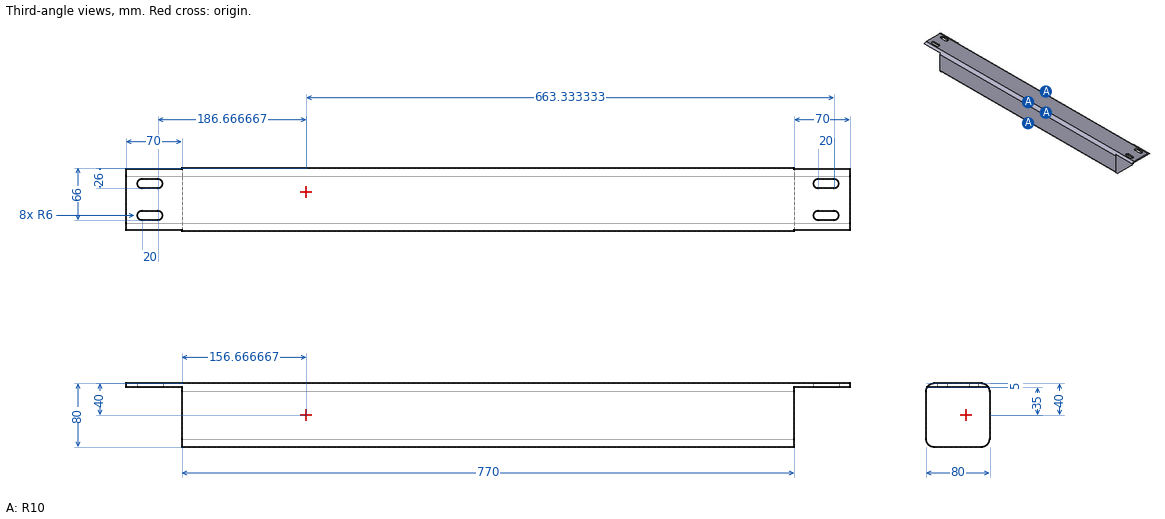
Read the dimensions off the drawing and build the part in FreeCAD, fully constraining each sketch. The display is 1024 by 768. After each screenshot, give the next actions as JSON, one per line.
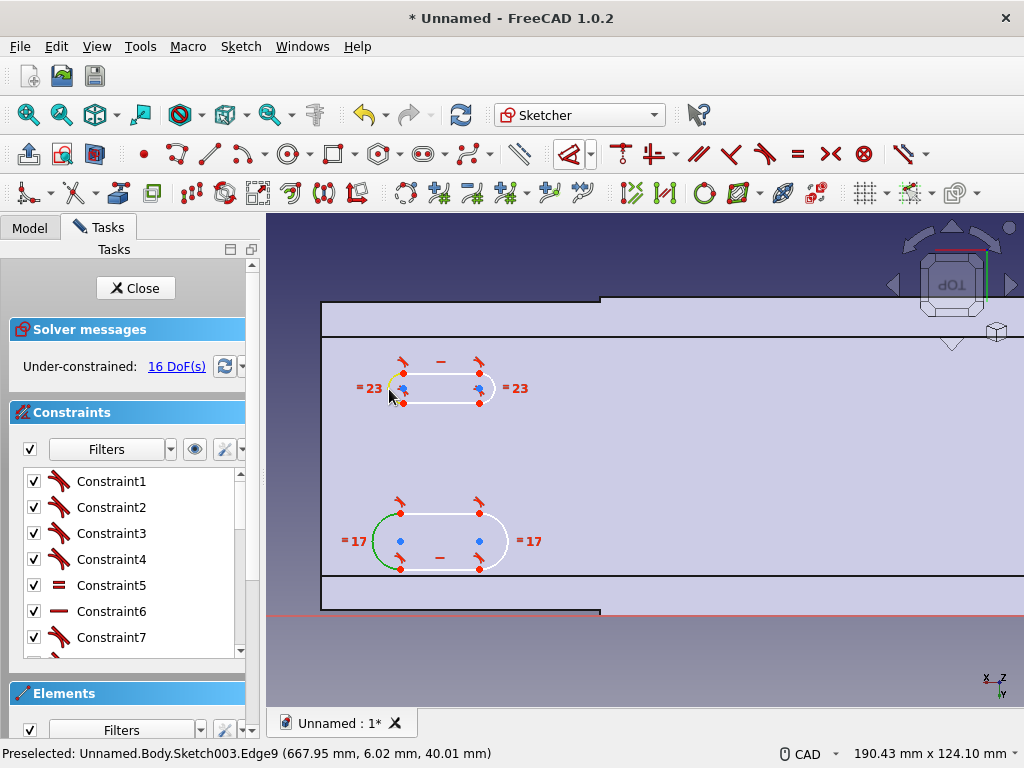
{"action": "left_click", "coordinate": [388, 388]}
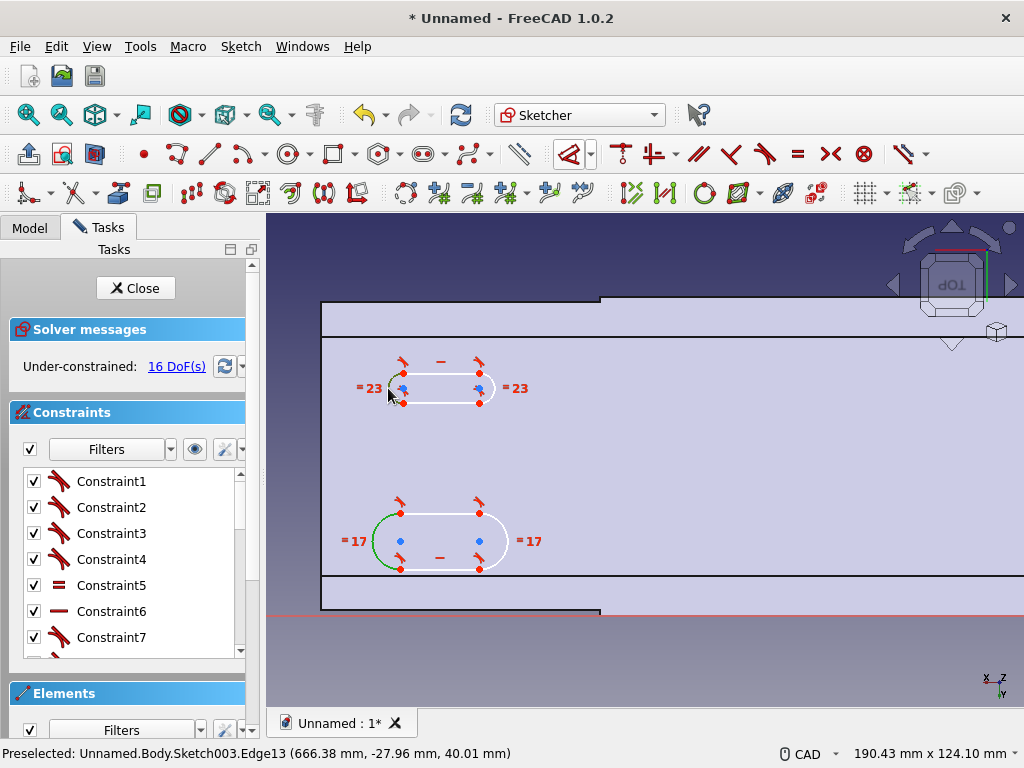
{"action": "left_click", "coordinate": [798, 154]}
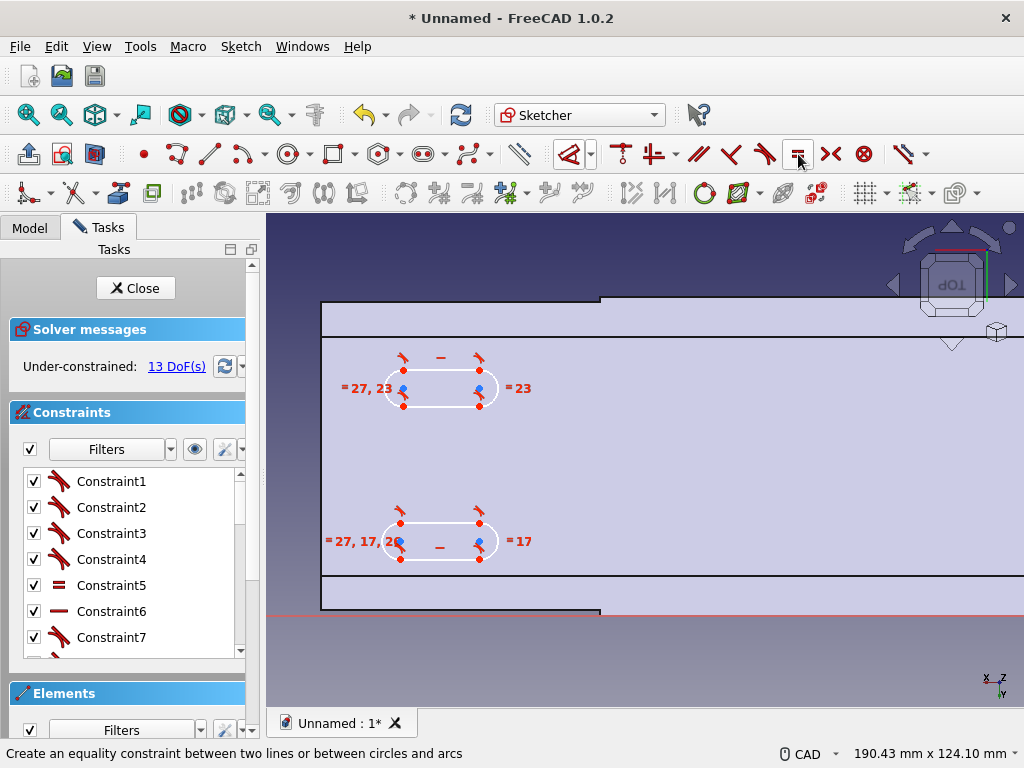
{"action": "scroll", "coordinate": [383, 457], "scroll_direction": "down", "scroll_amount": 11}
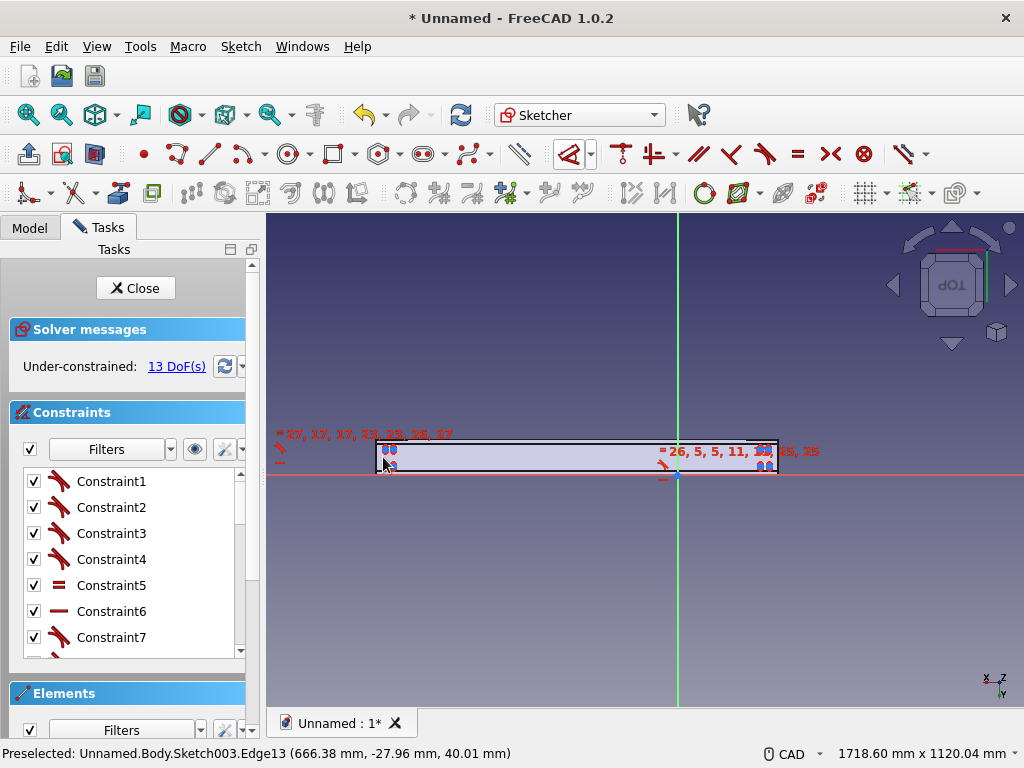
{"action": "scroll", "coordinate": [758, 448], "scroll_direction": "up", "scroll_amount": 14}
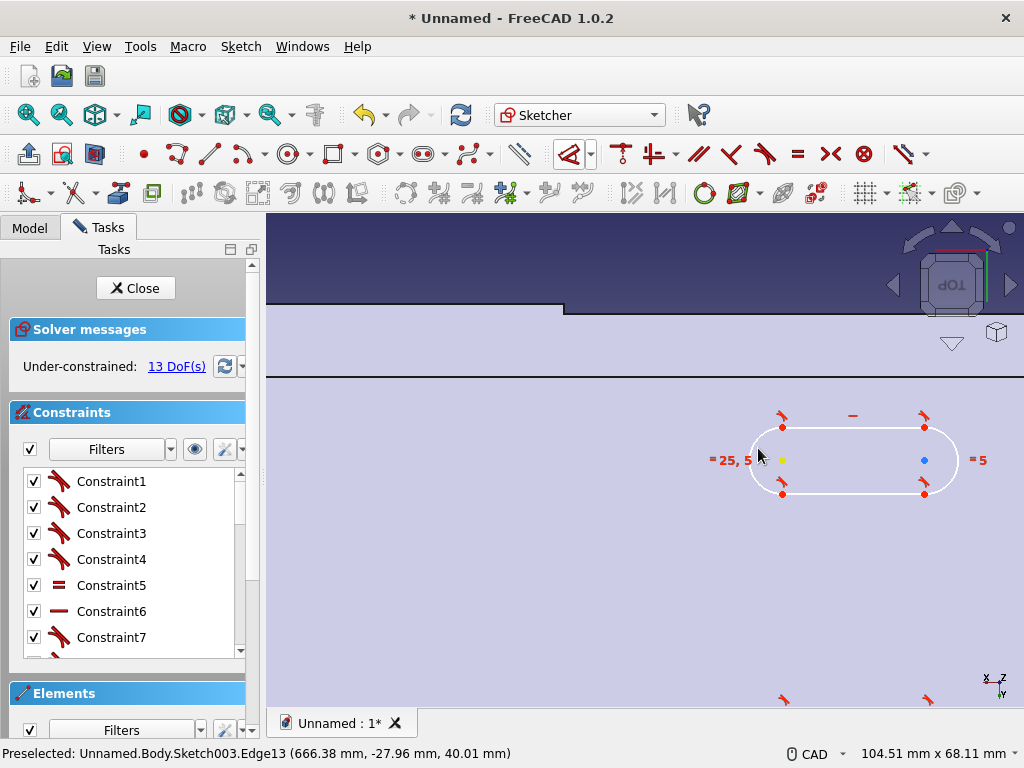
{"action": "left_click", "coordinate": [756, 441]}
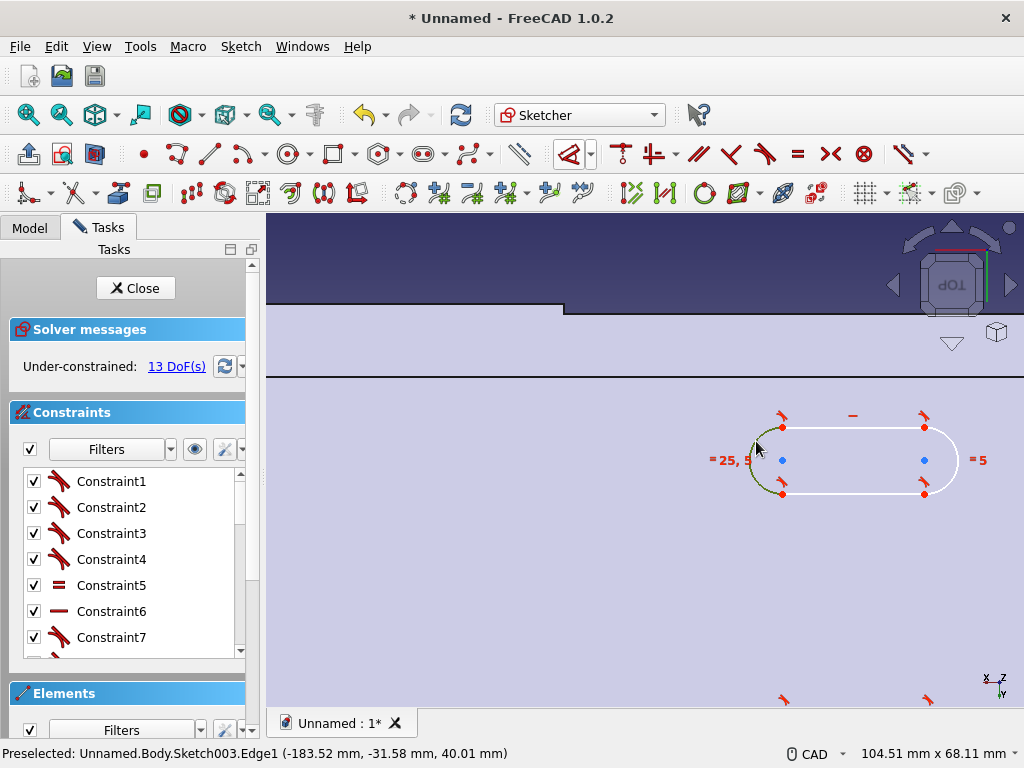
{"action": "left_click", "coordinate": [590, 154]}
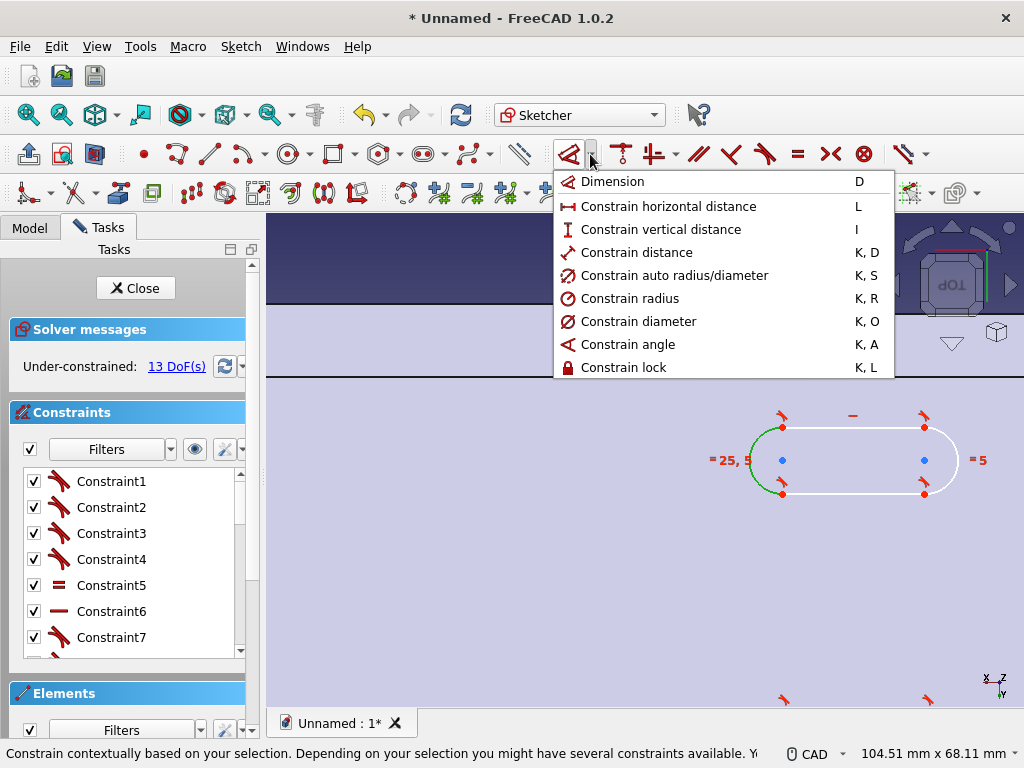
{"action": "left_click", "coordinate": [724, 298]}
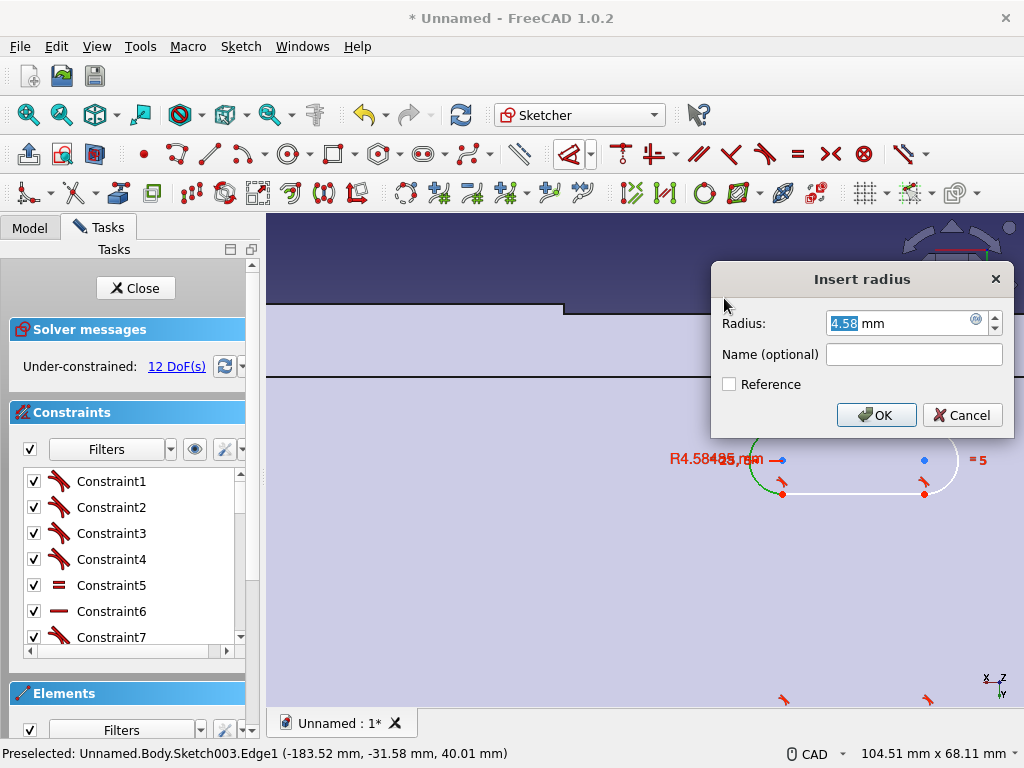
{"action": "type", "text": "6"}
{"action": "key", "text": "Return"}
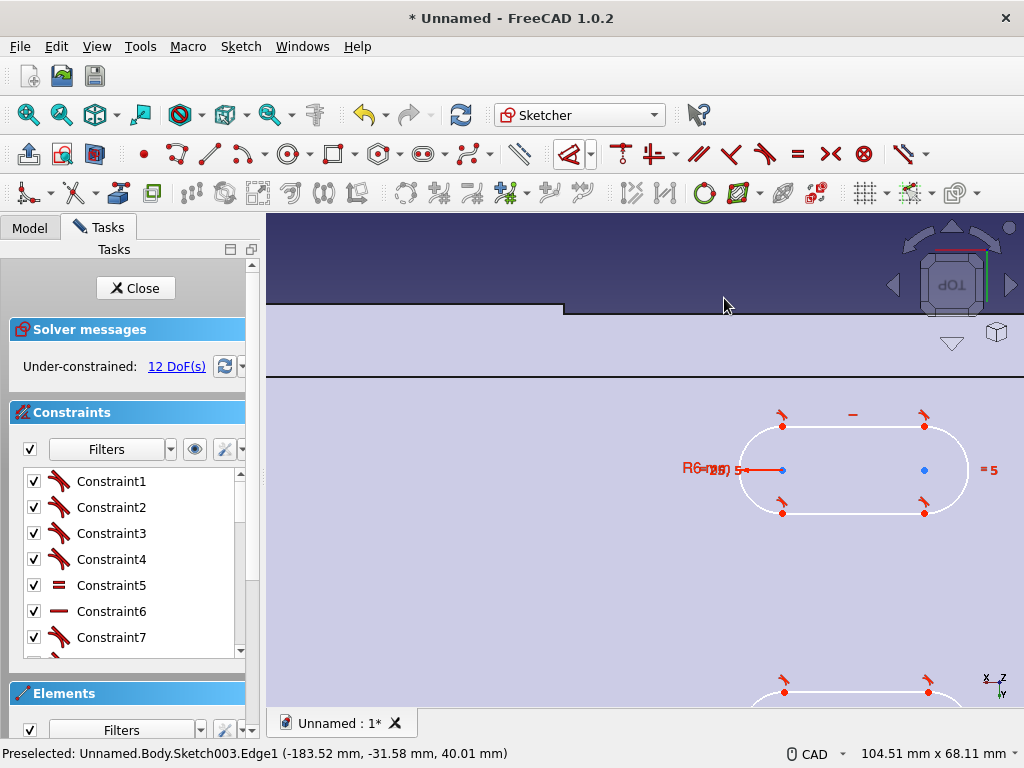
{"action": "scroll", "coordinate": [758, 448], "scroll_direction": "down", "scroll_amount": 14}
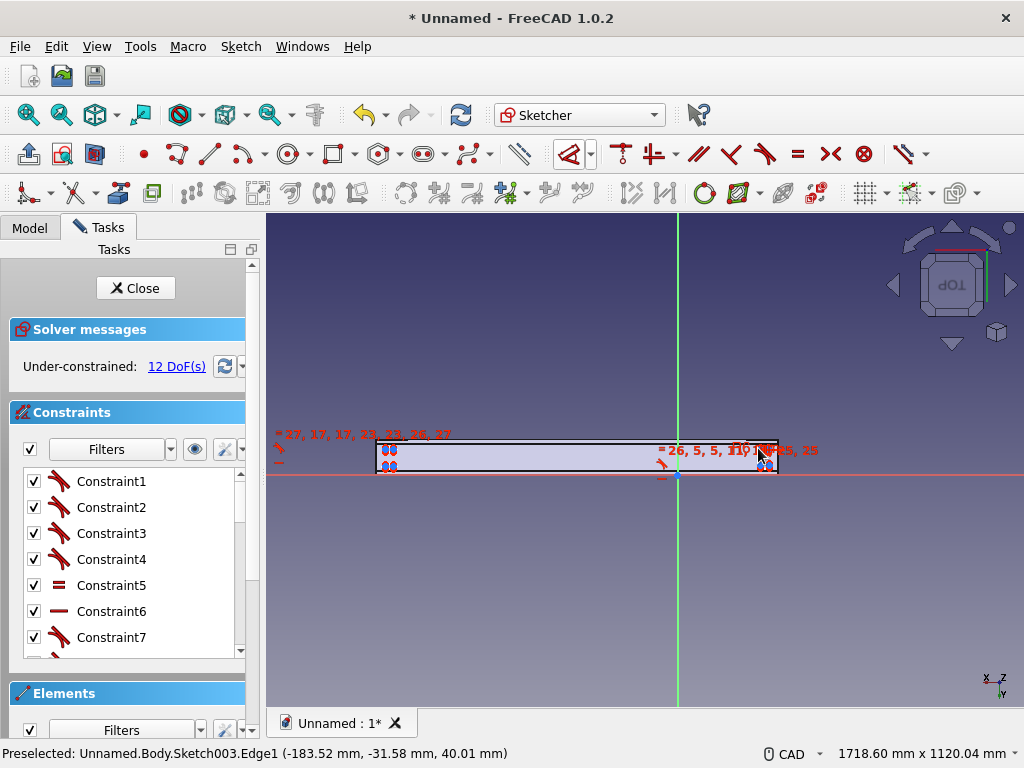
{"action": "scroll", "coordinate": [763, 447], "scroll_direction": "up", "scroll_amount": 9}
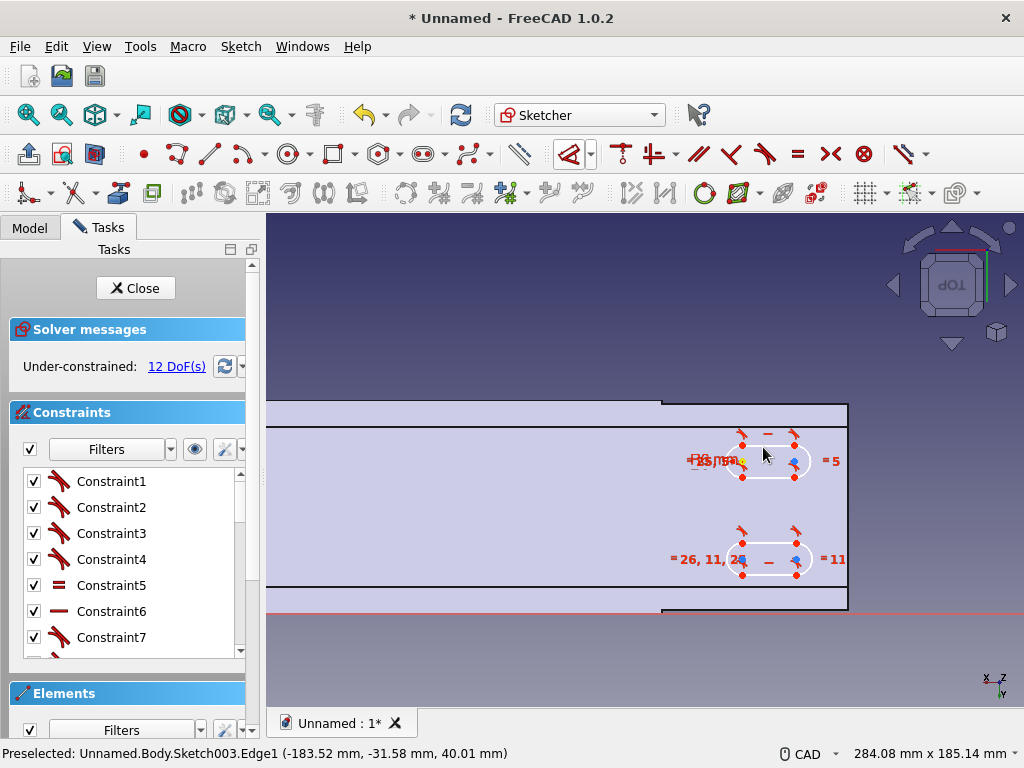
{"action": "left_click", "coordinate": [758, 446]}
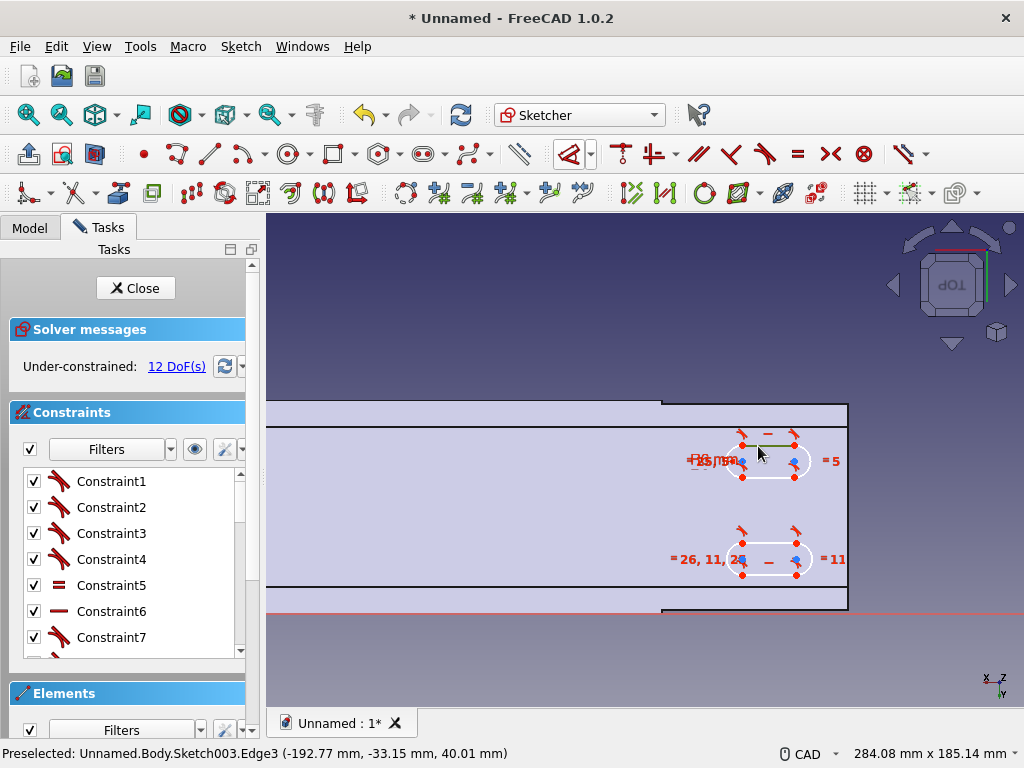
{"action": "key", "text": "l"}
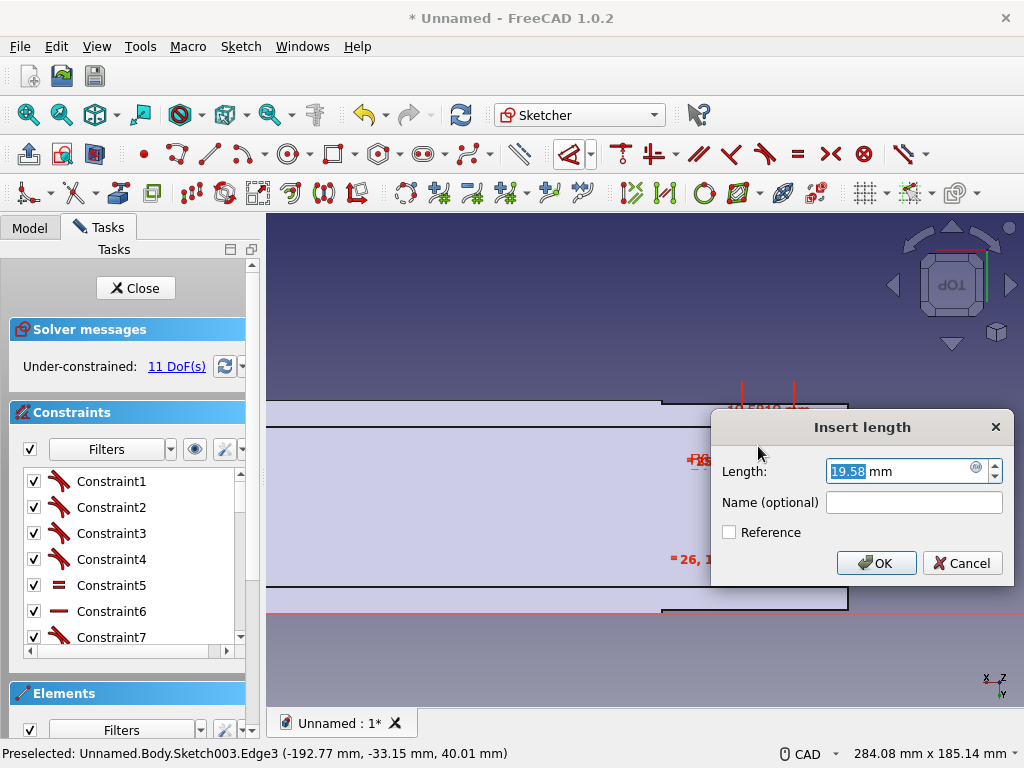
{"action": "type", "text": "20"}
{"action": "key", "text": "Return"}